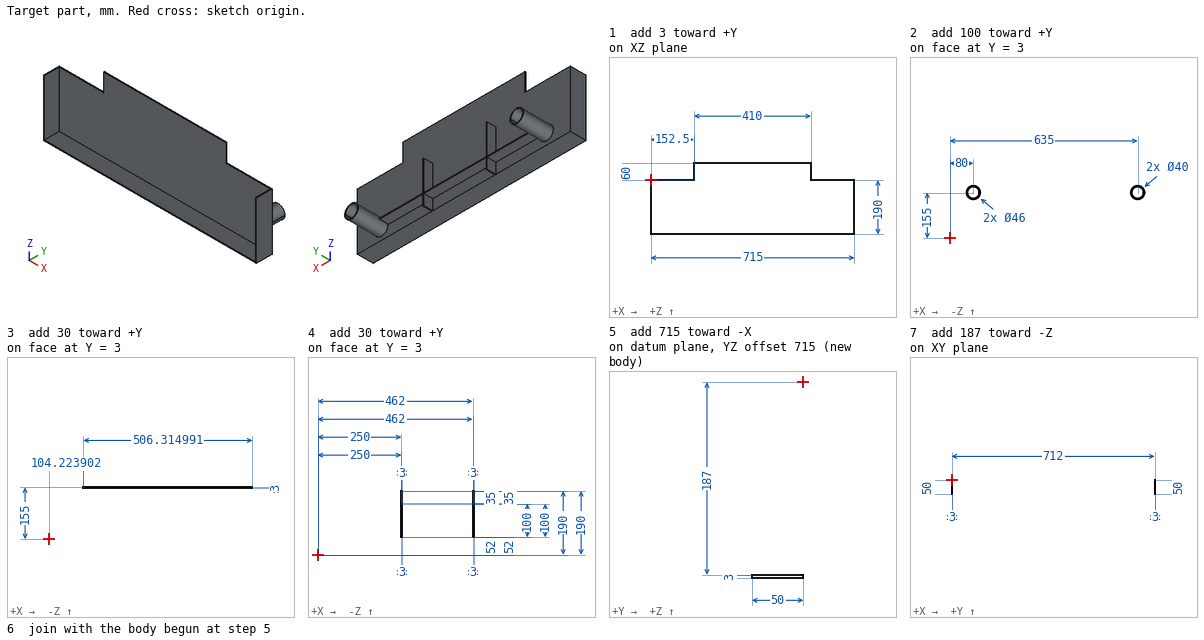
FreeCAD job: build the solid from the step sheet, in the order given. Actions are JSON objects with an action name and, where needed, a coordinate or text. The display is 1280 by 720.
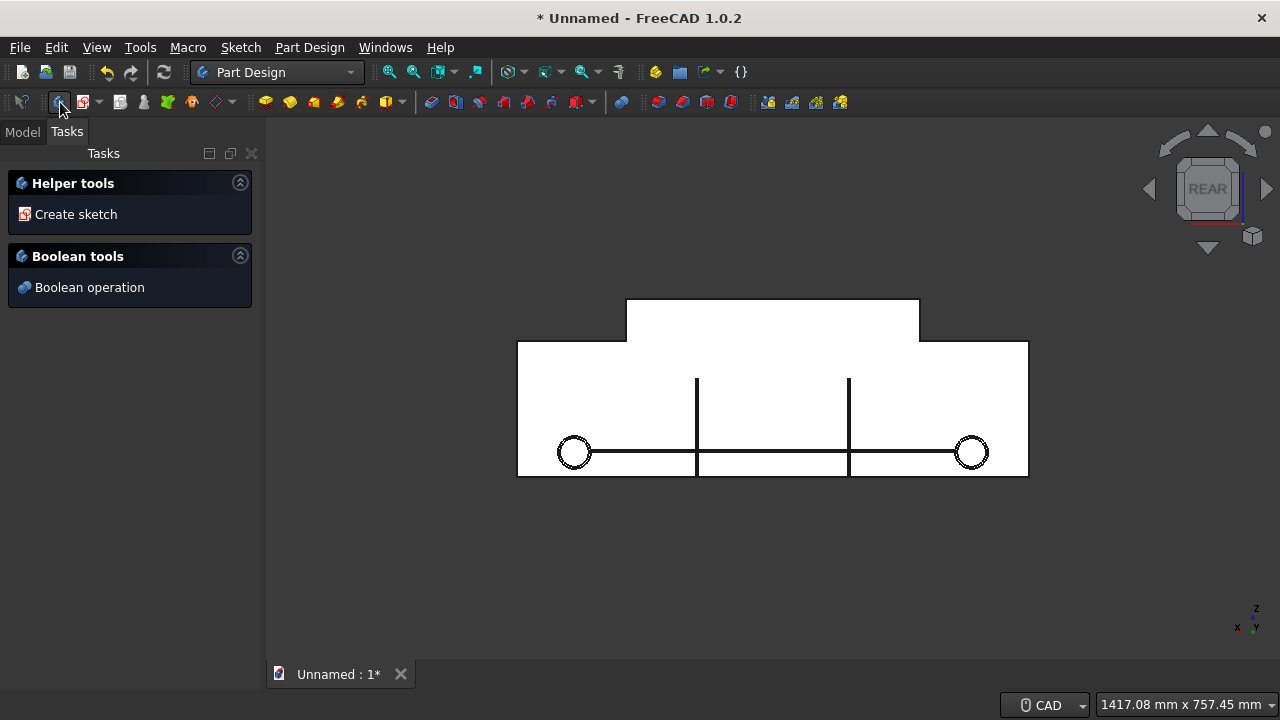
{"action": "left_click", "coordinate": [23, 131]}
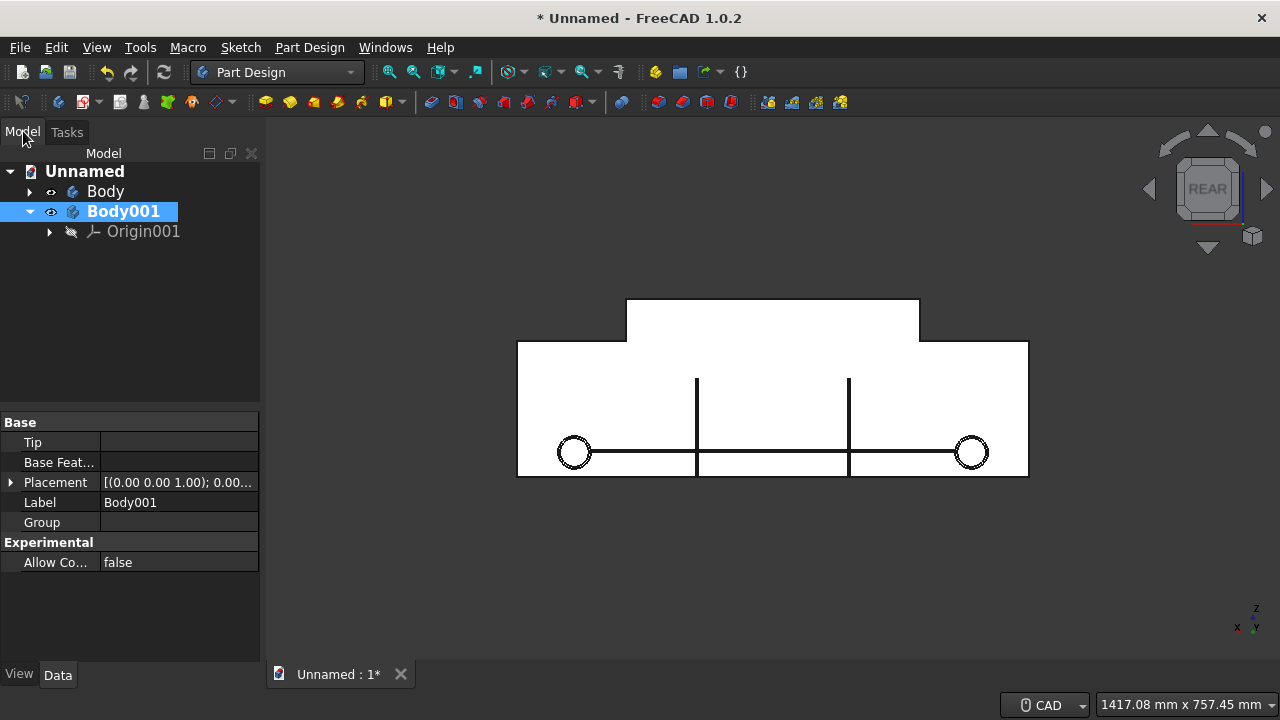
{"action": "left_click", "coordinate": [50, 232]}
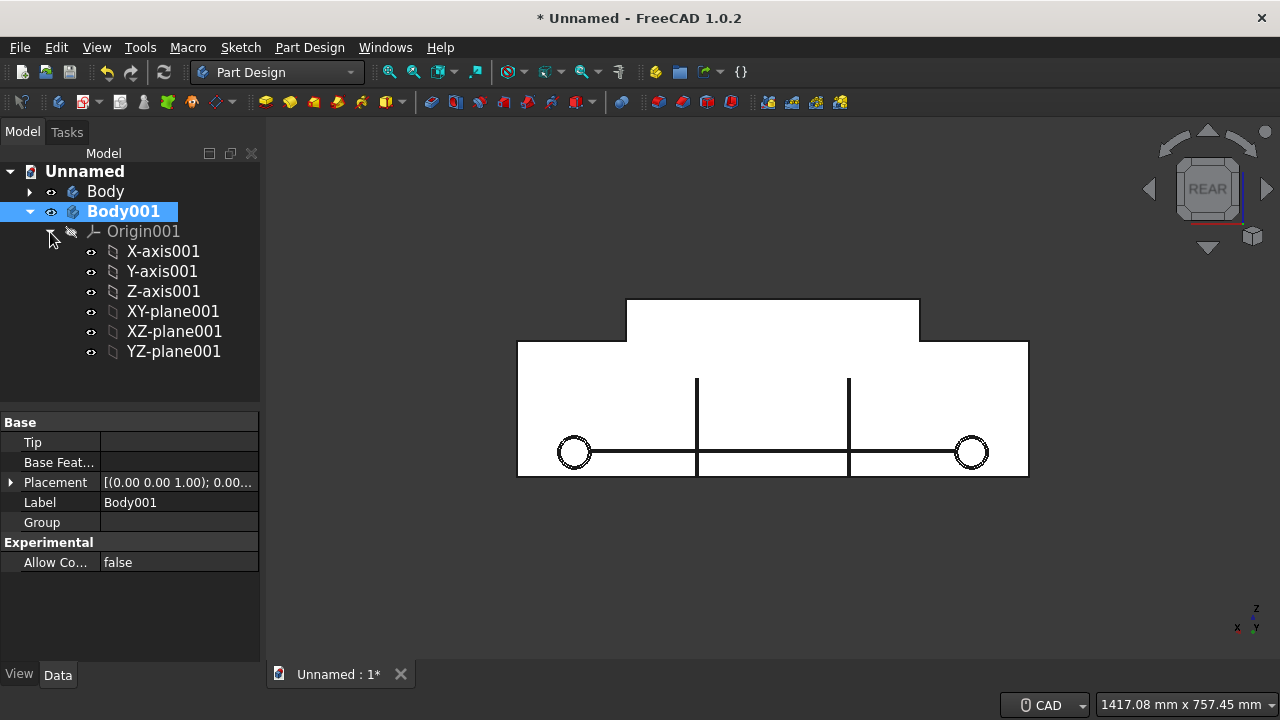
{"action": "left_click", "coordinate": [136, 352]}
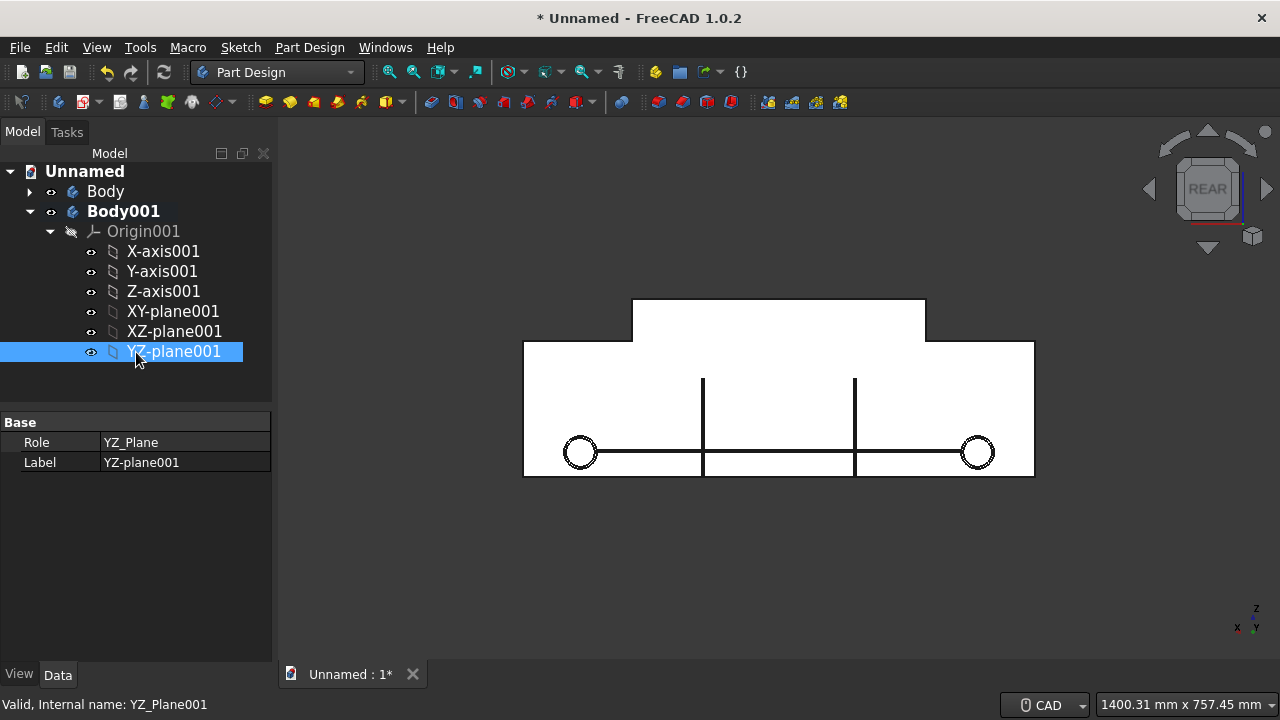
{"action": "left_click", "coordinate": [216, 102]}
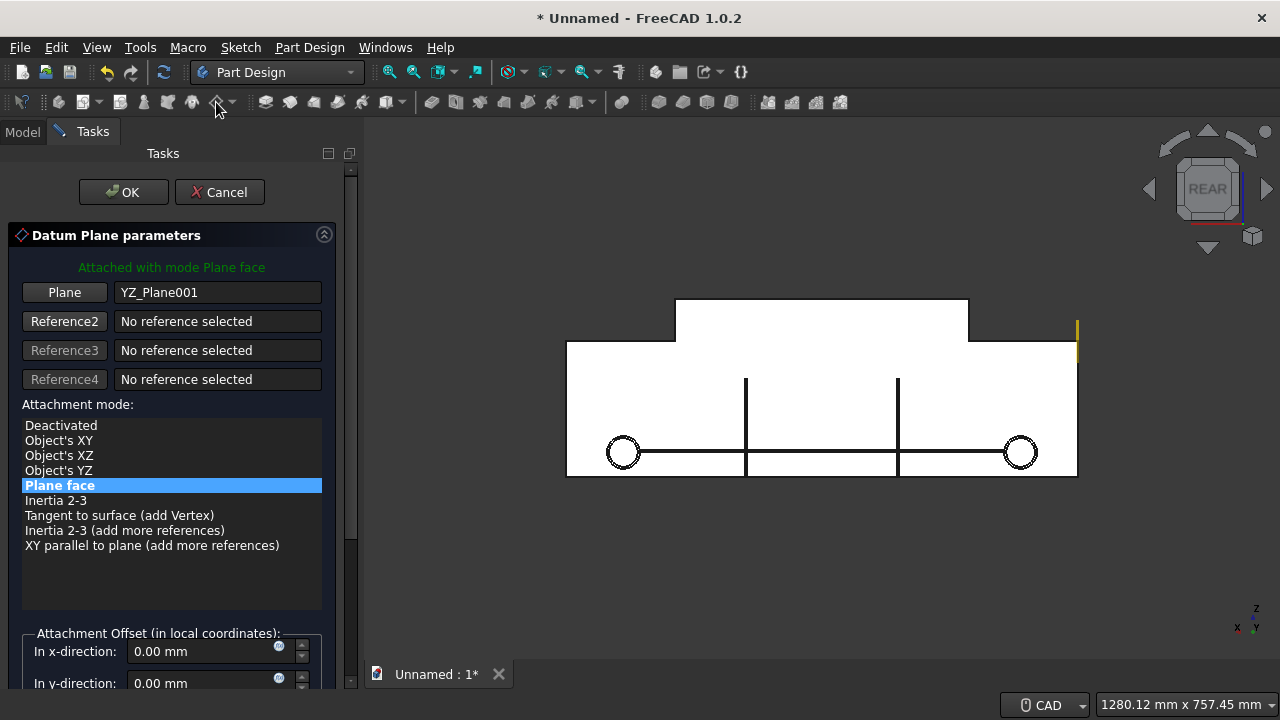
{"action": "scroll", "coordinate": [351, 426], "scroll_direction": "down", "scroll_amount": 2}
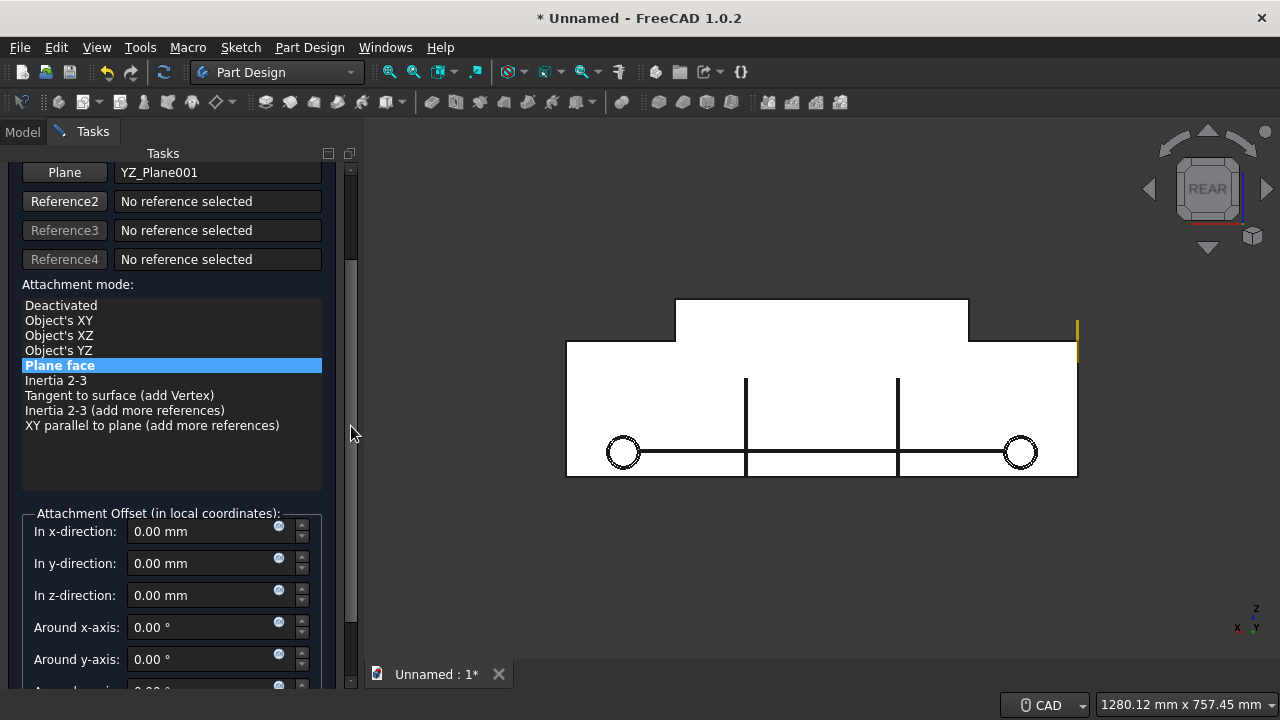
{"action": "triple_click", "coordinate": [210, 595]}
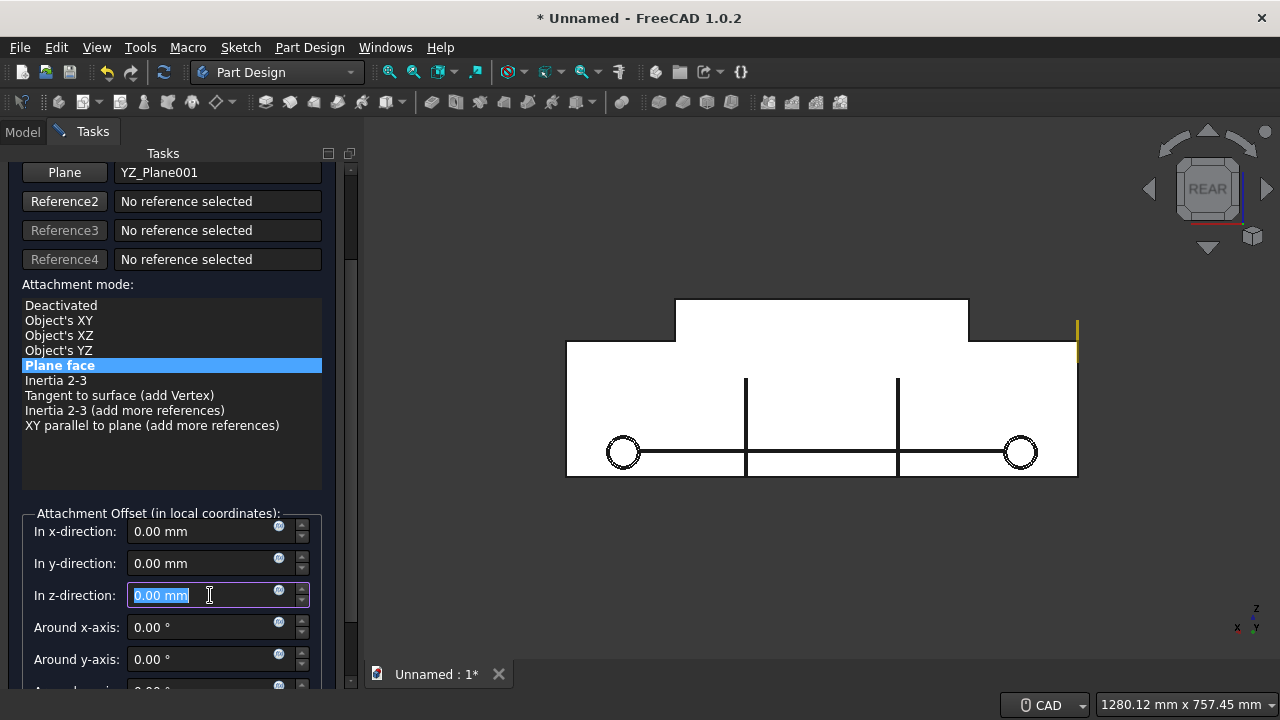
{"action": "type", "text": "715"}
{"action": "key", "text": "Tab"}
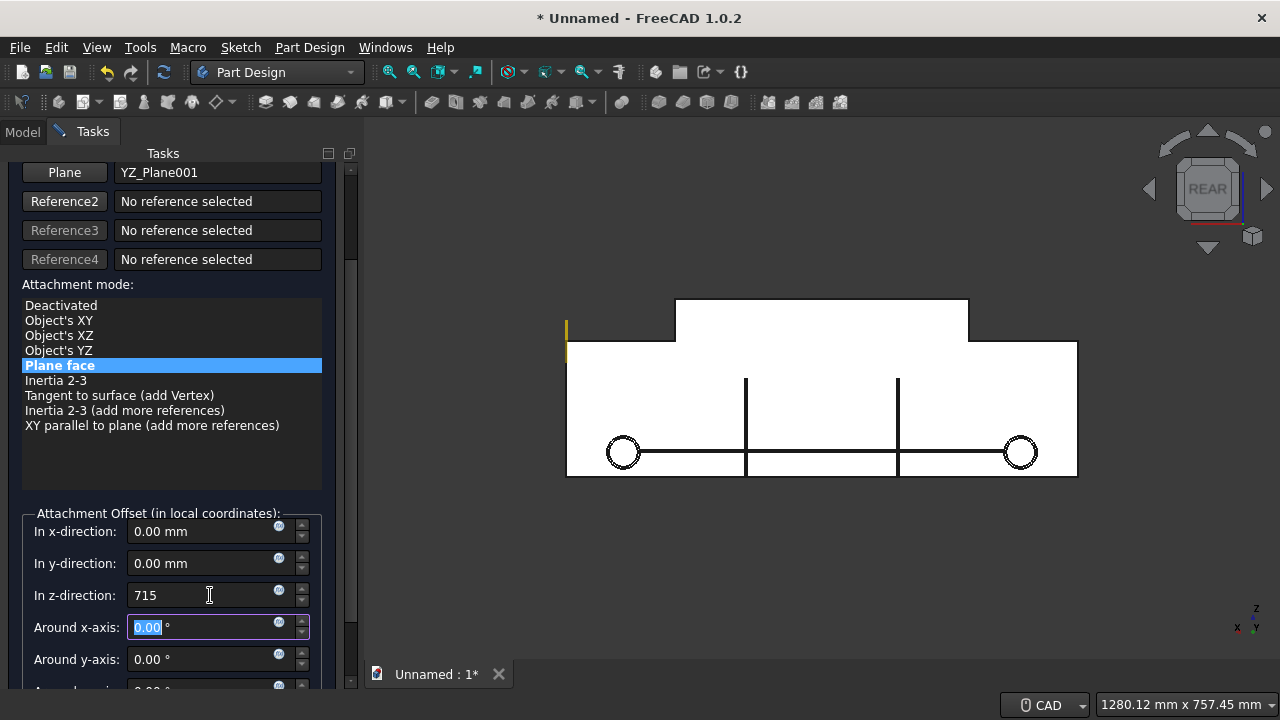
{"action": "scroll", "coordinate": [351, 426], "scroll_direction": "up", "scroll_amount": 3}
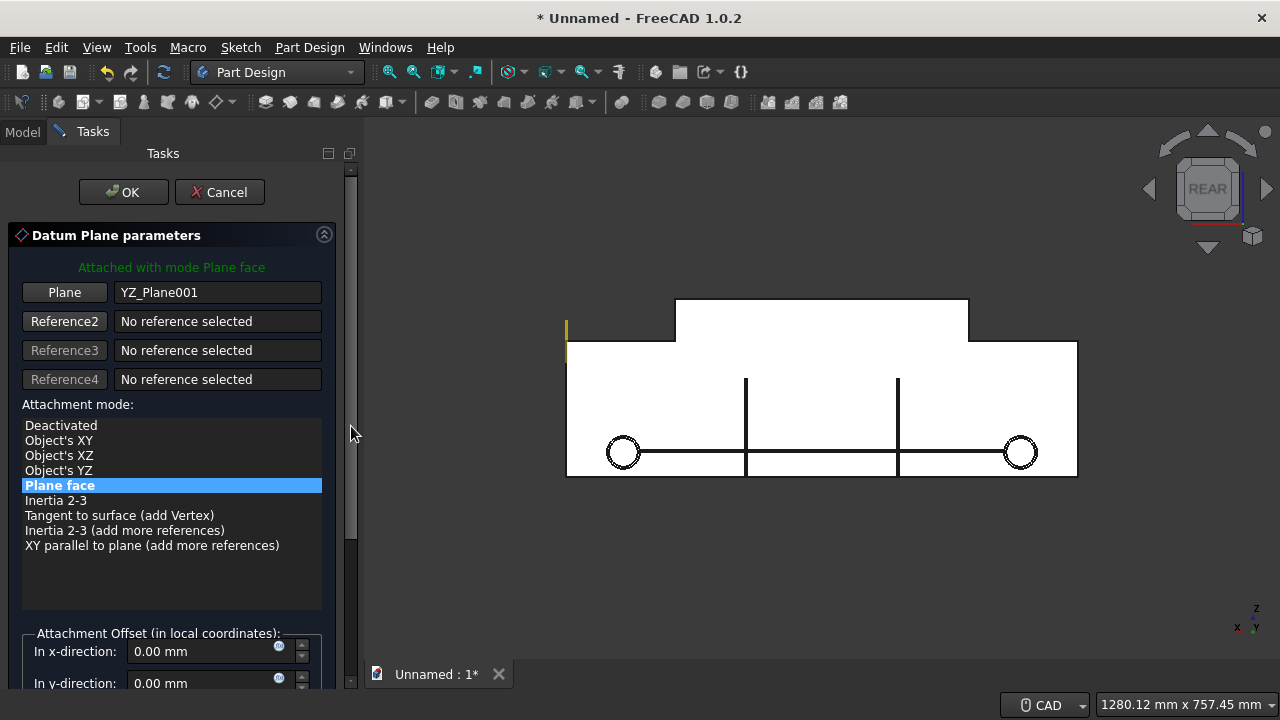
{"action": "left_click", "coordinate": [124, 192]}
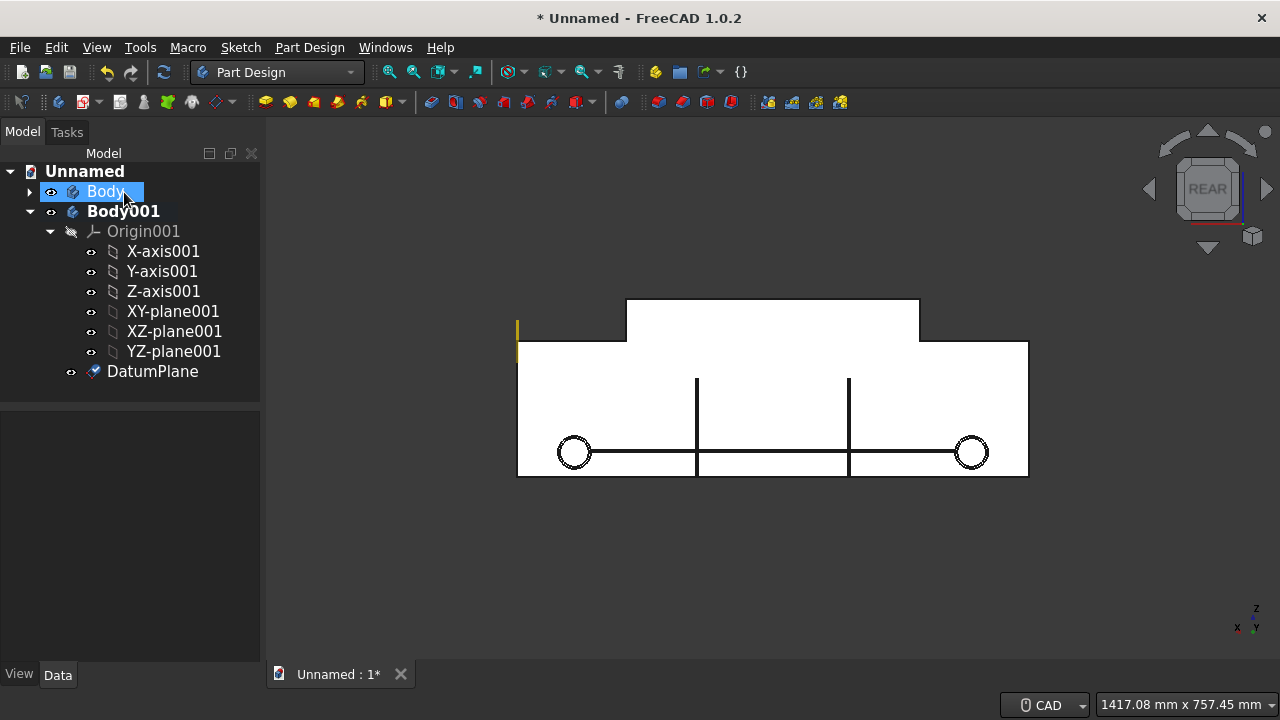
{"action": "left_click", "coordinate": [116, 372]}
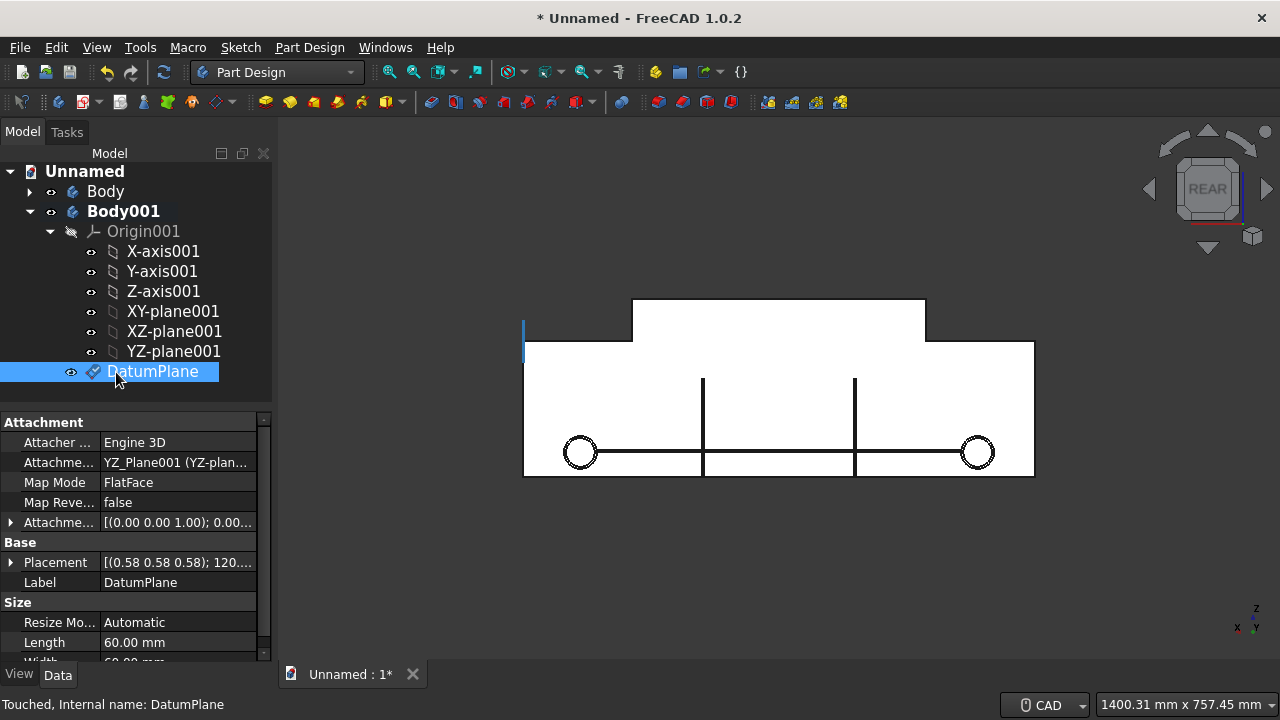
{"action": "left_click", "coordinate": [84, 102]}